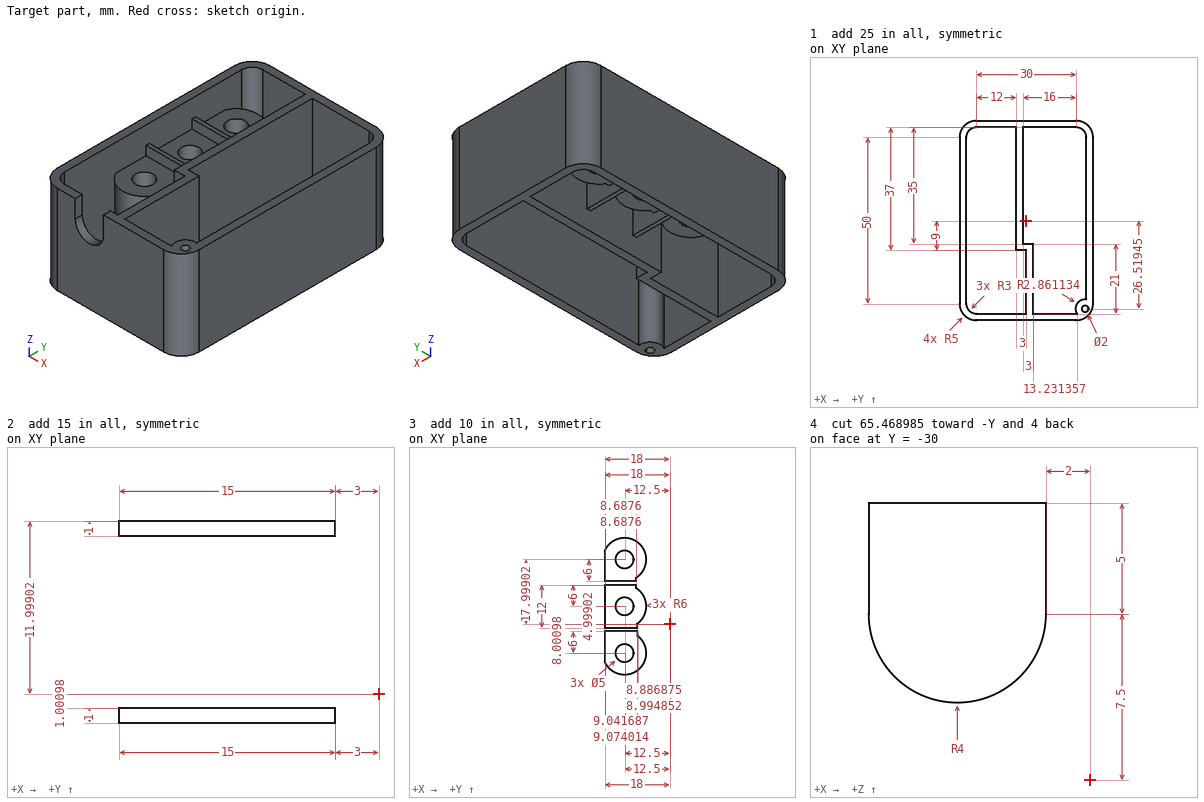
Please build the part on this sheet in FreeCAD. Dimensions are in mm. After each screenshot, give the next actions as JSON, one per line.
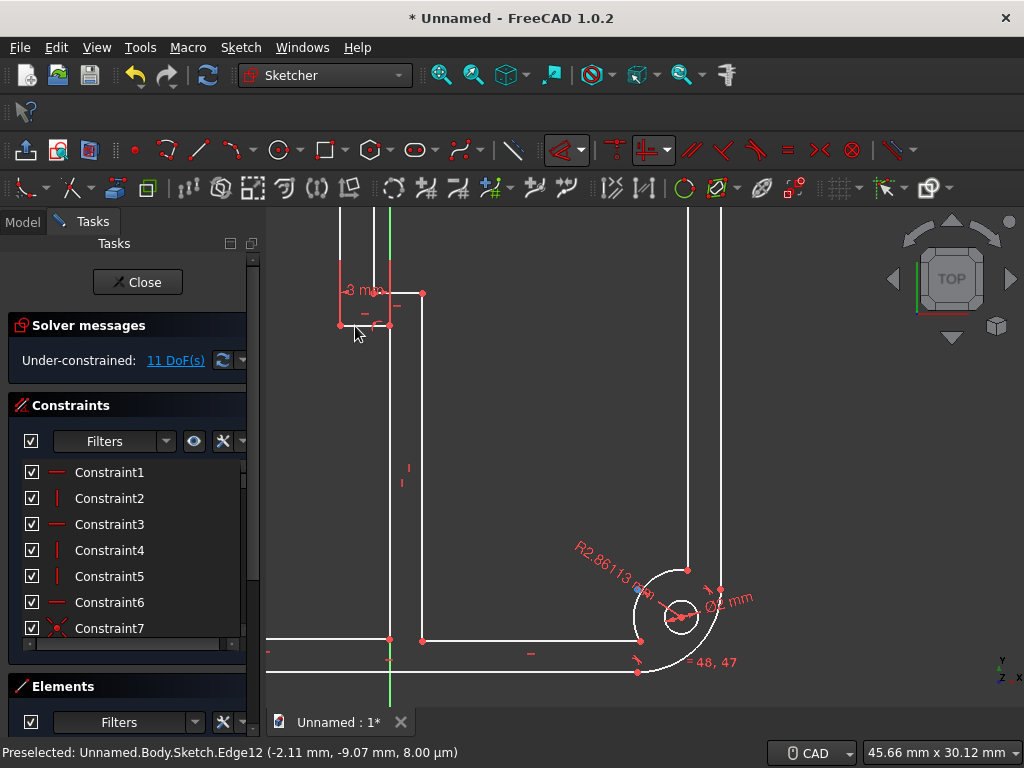
{"action": "left_click", "coordinate": [408, 293]}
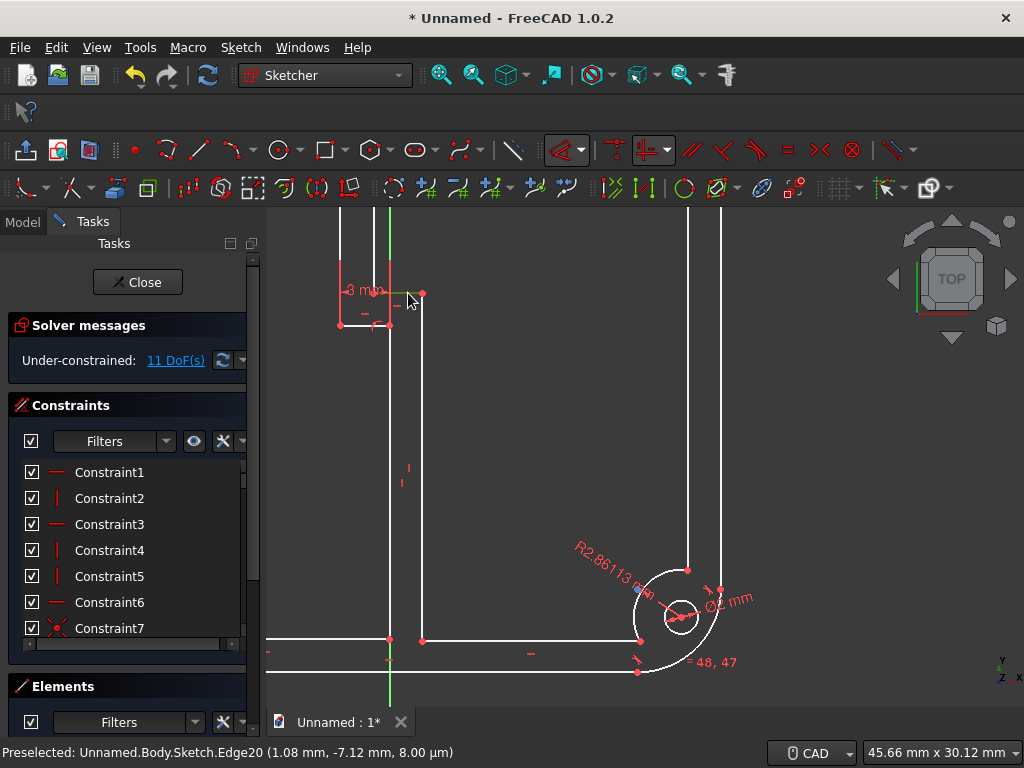
{"action": "key", "text": "l"}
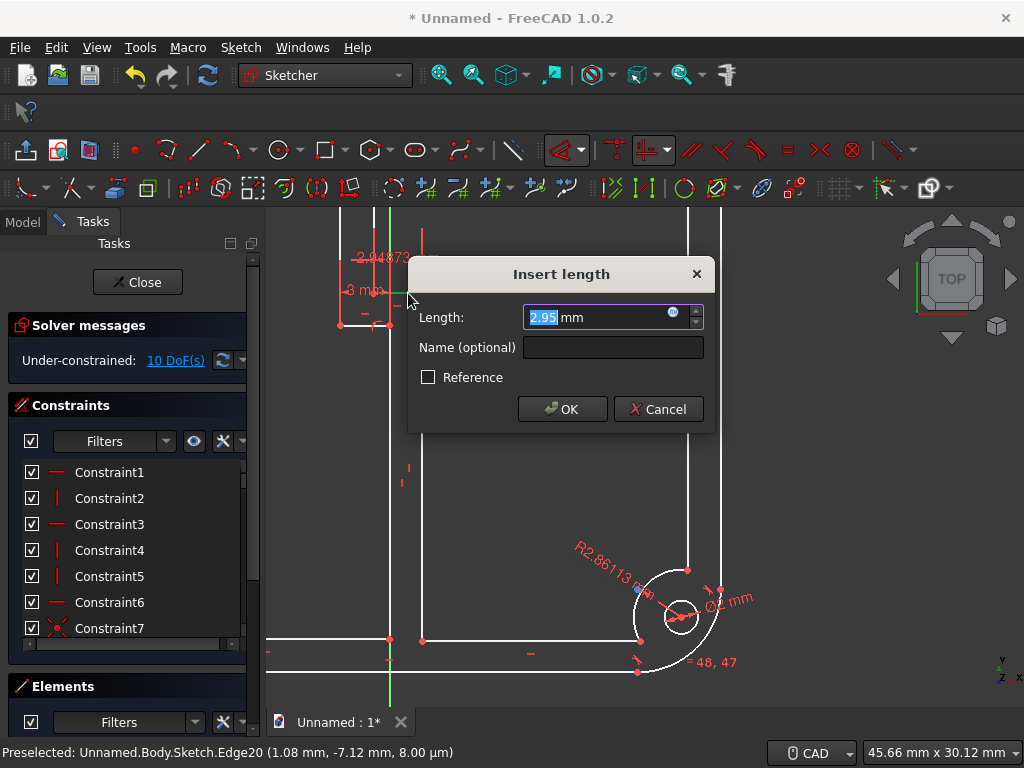
{"action": "type", "text": "3"}
{"action": "key", "text": "Return"}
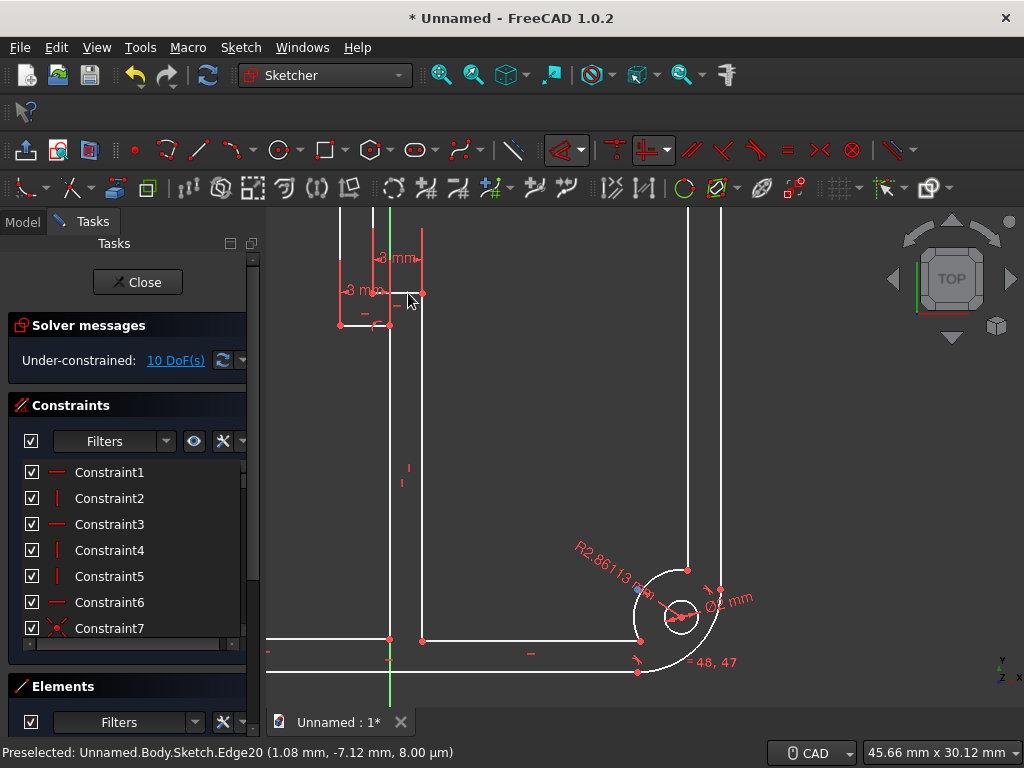
{"action": "scroll", "coordinate": [657, 579], "scroll_direction": "down", "scroll_amount": 6}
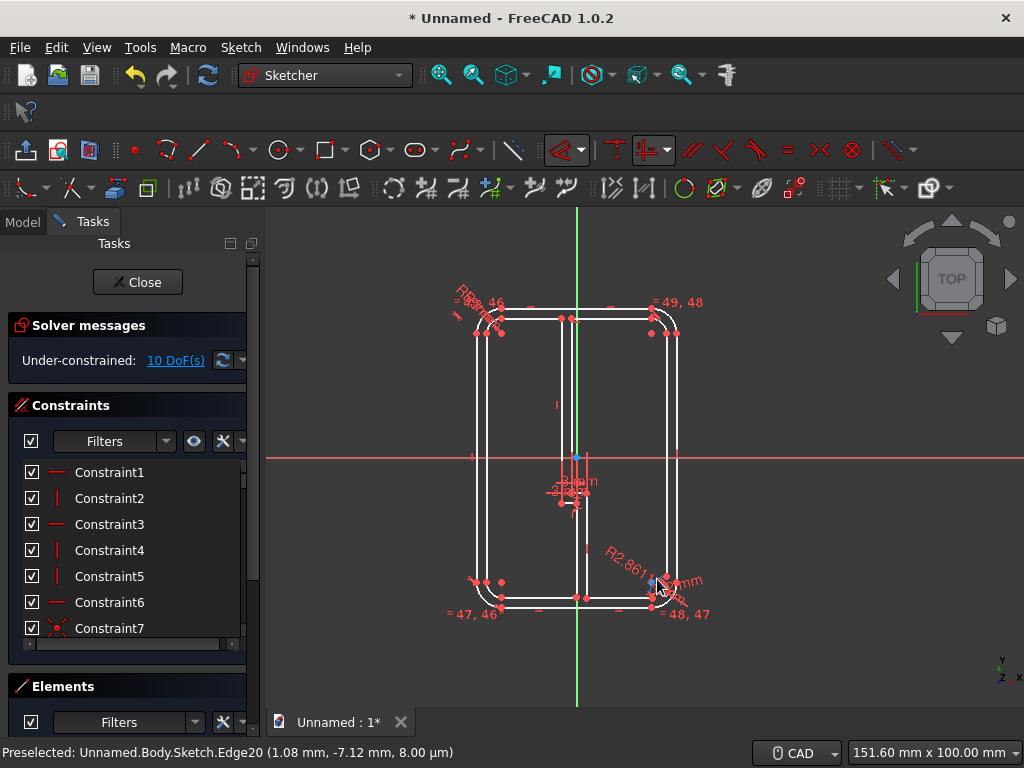
{"action": "scroll", "coordinate": [607, 309], "scroll_direction": "up", "scroll_amount": 2}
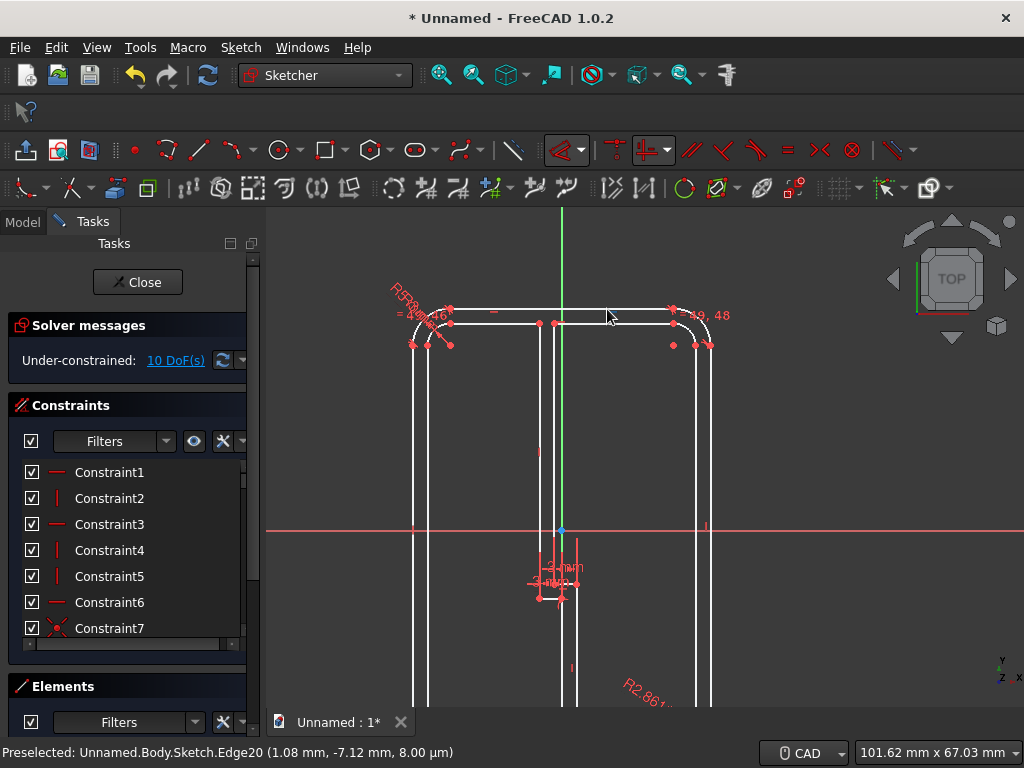
{"action": "left_click", "coordinate": [606, 309]}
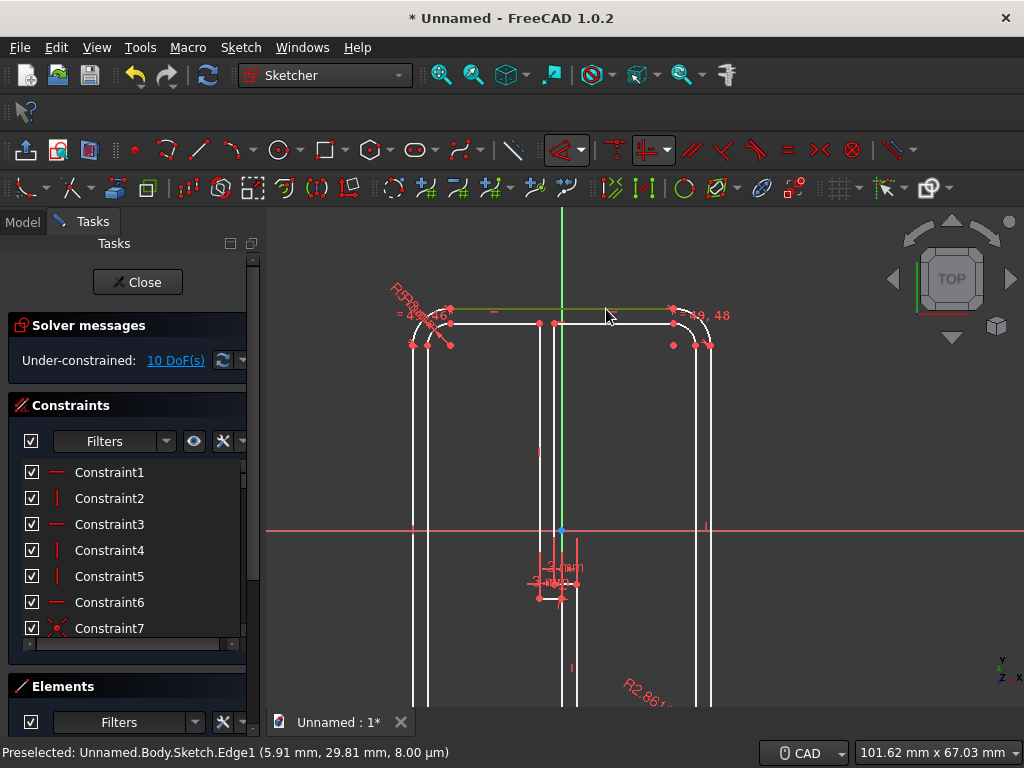
{"action": "key", "text": "l"}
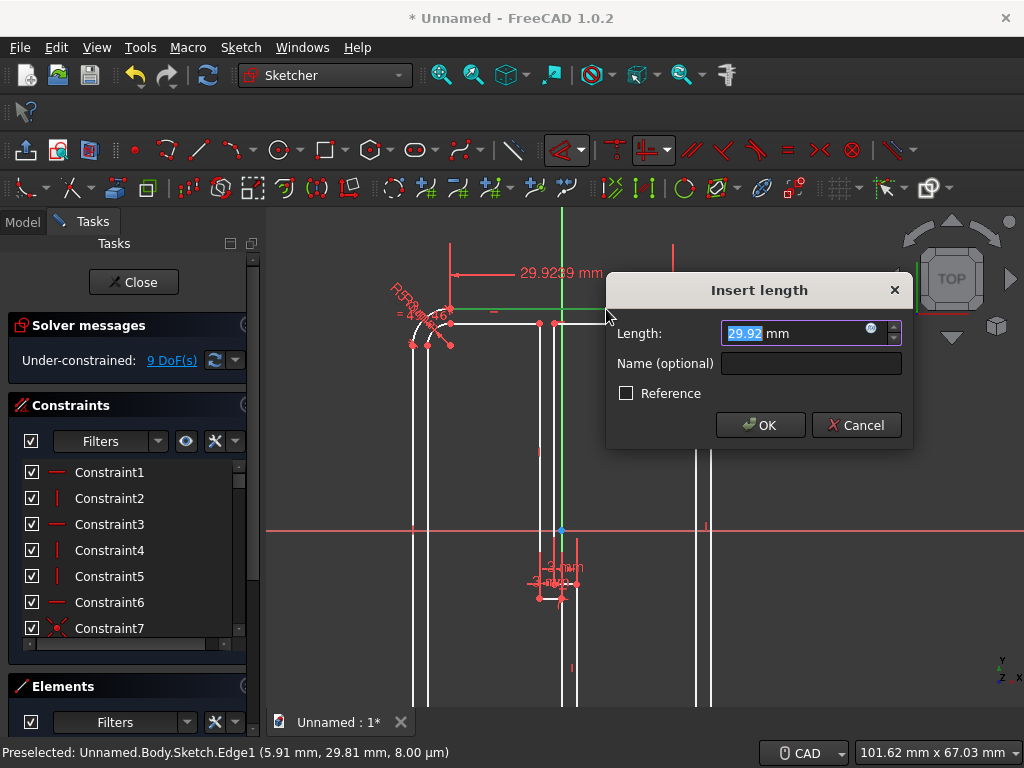
{"action": "type", "text": "30"}
{"action": "key", "text": "Return"}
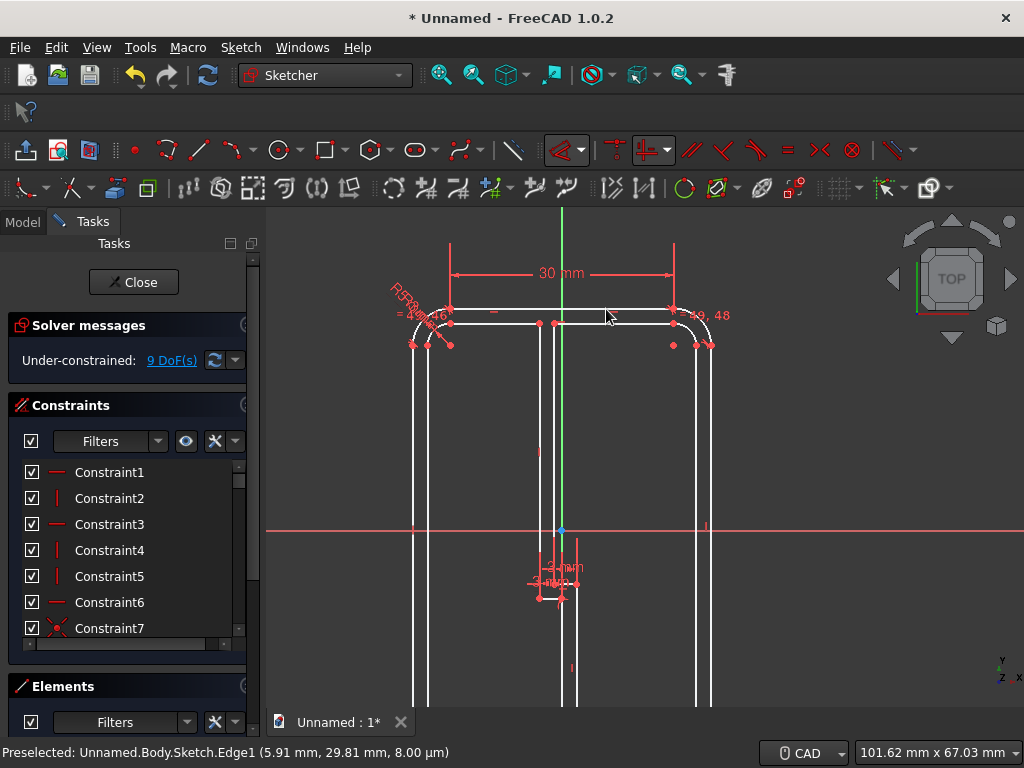
{"action": "left_click", "coordinate": [413, 457]}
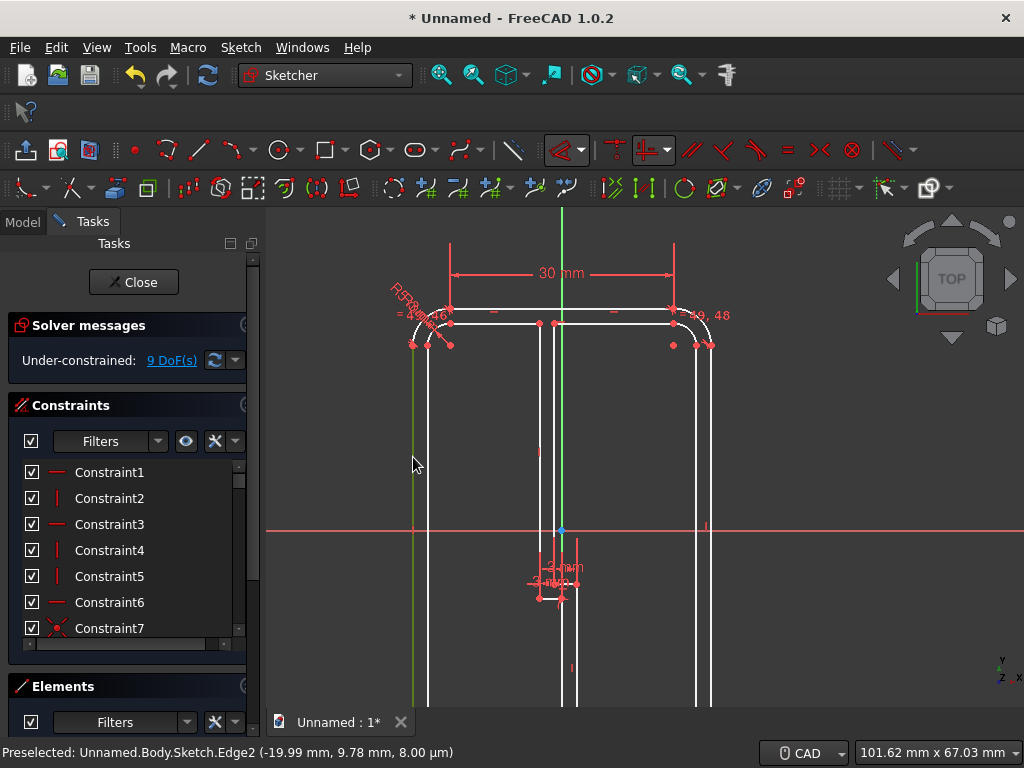
{"action": "left_click", "coordinate": [584, 150]}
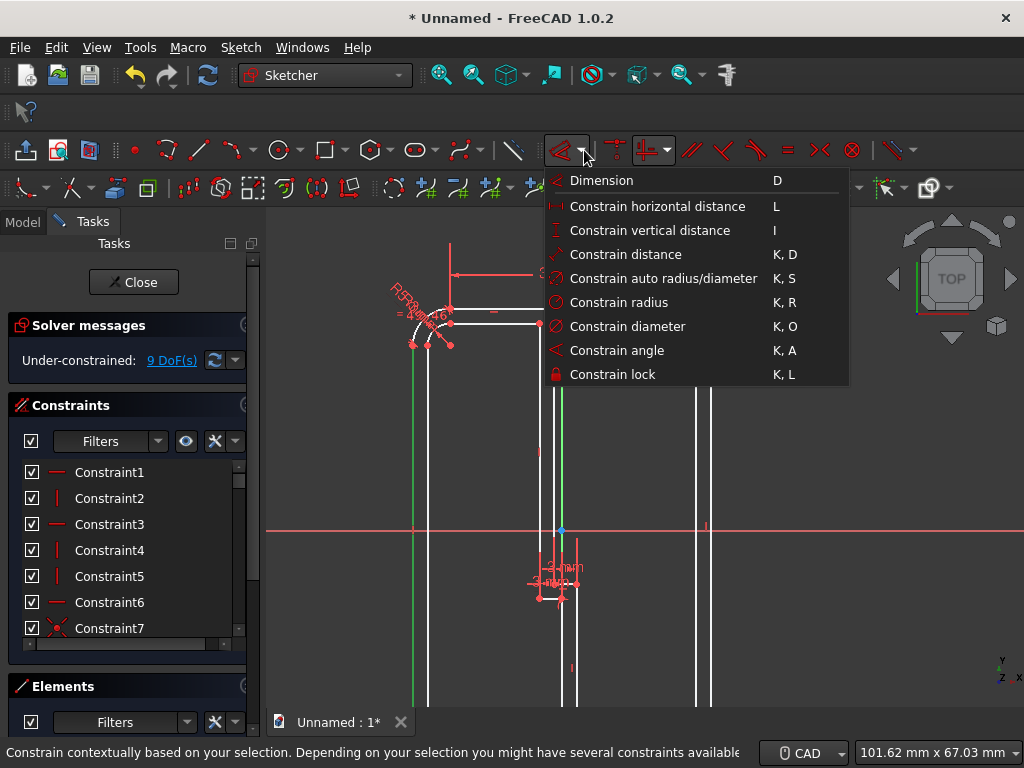
{"action": "left_click", "coordinate": [697, 230]}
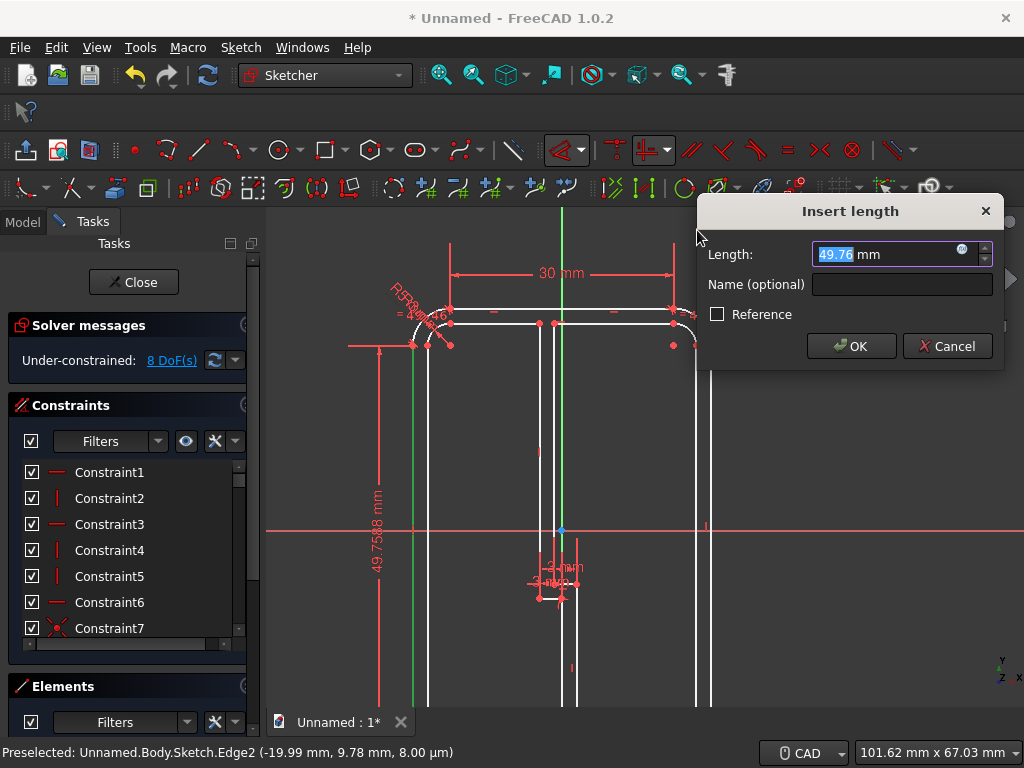
{"action": "type", "text": "50"}
{"action": "key", "text": "Return"}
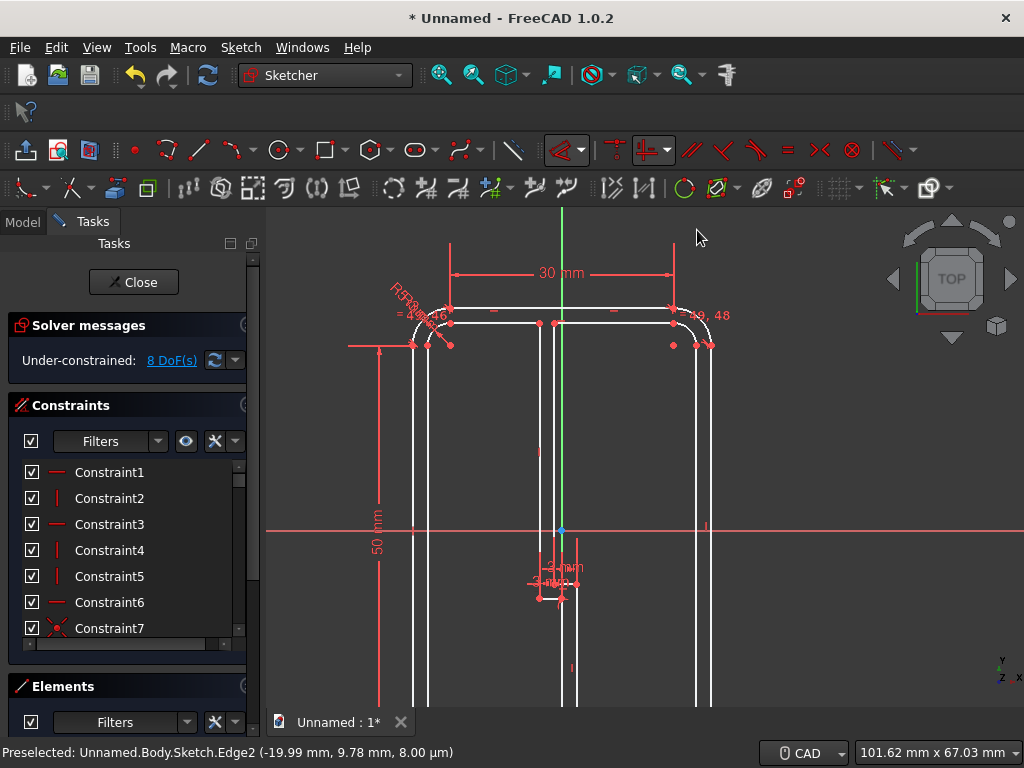
{"action": "left_click", "coordinate": [477, 323]}